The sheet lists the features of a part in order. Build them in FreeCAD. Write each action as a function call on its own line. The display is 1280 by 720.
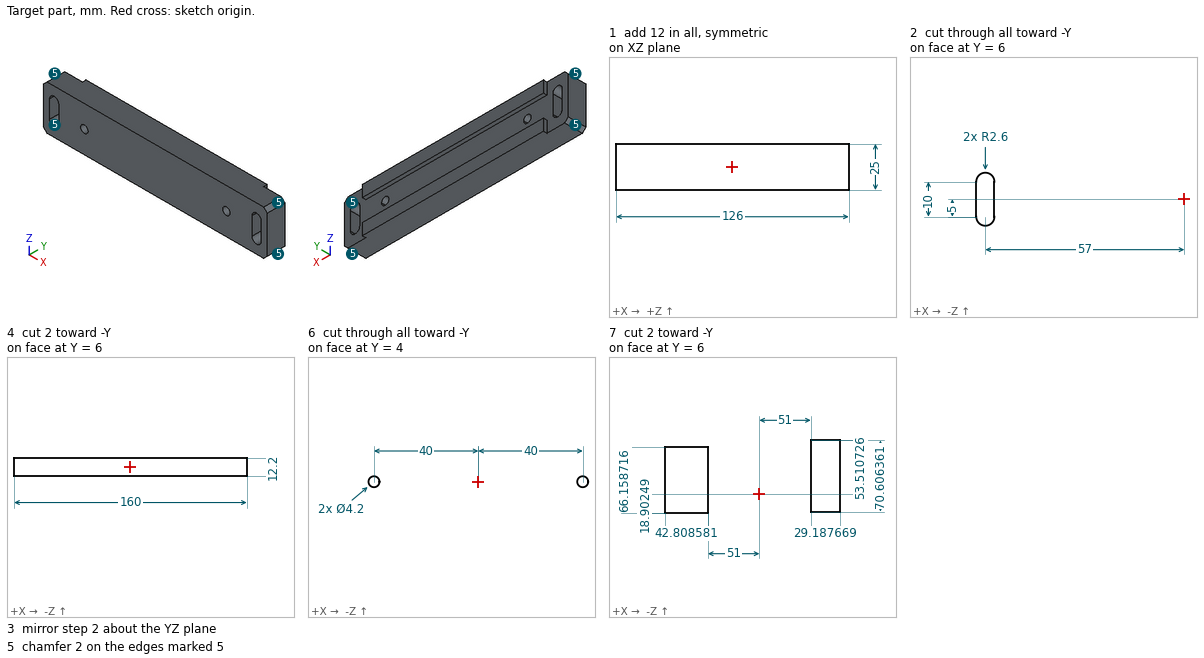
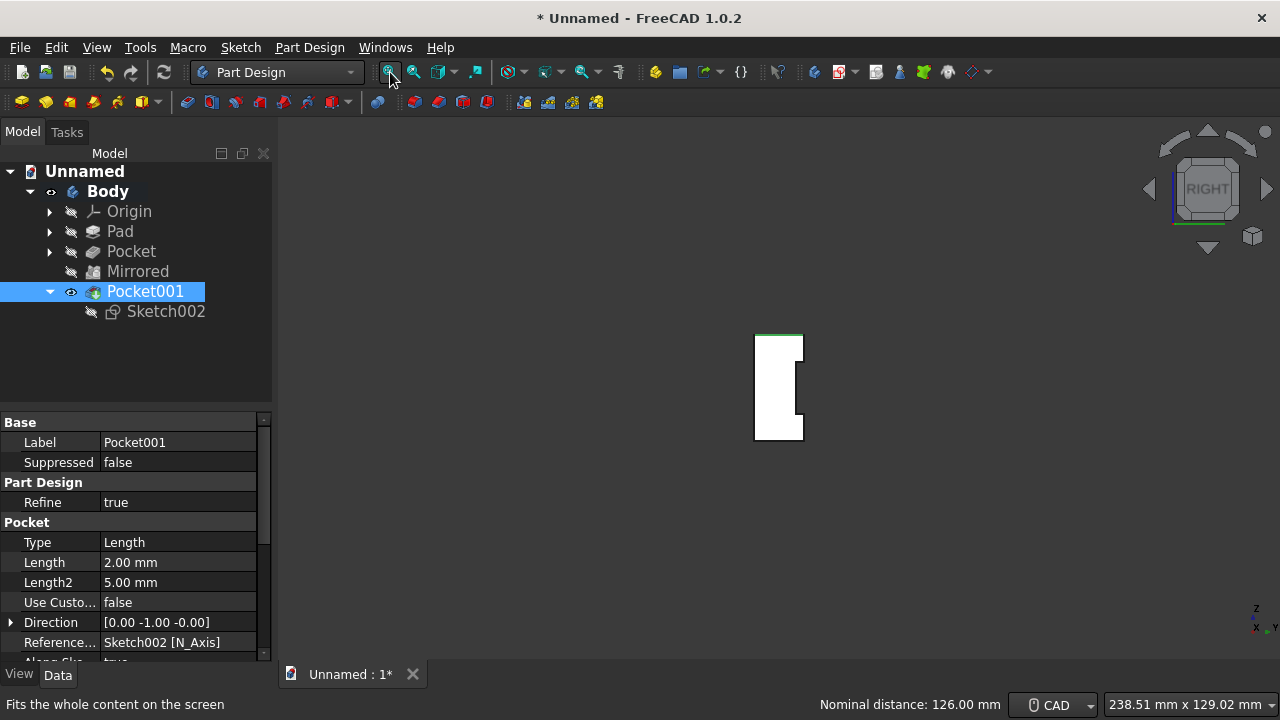
click(779, 440, ctrl)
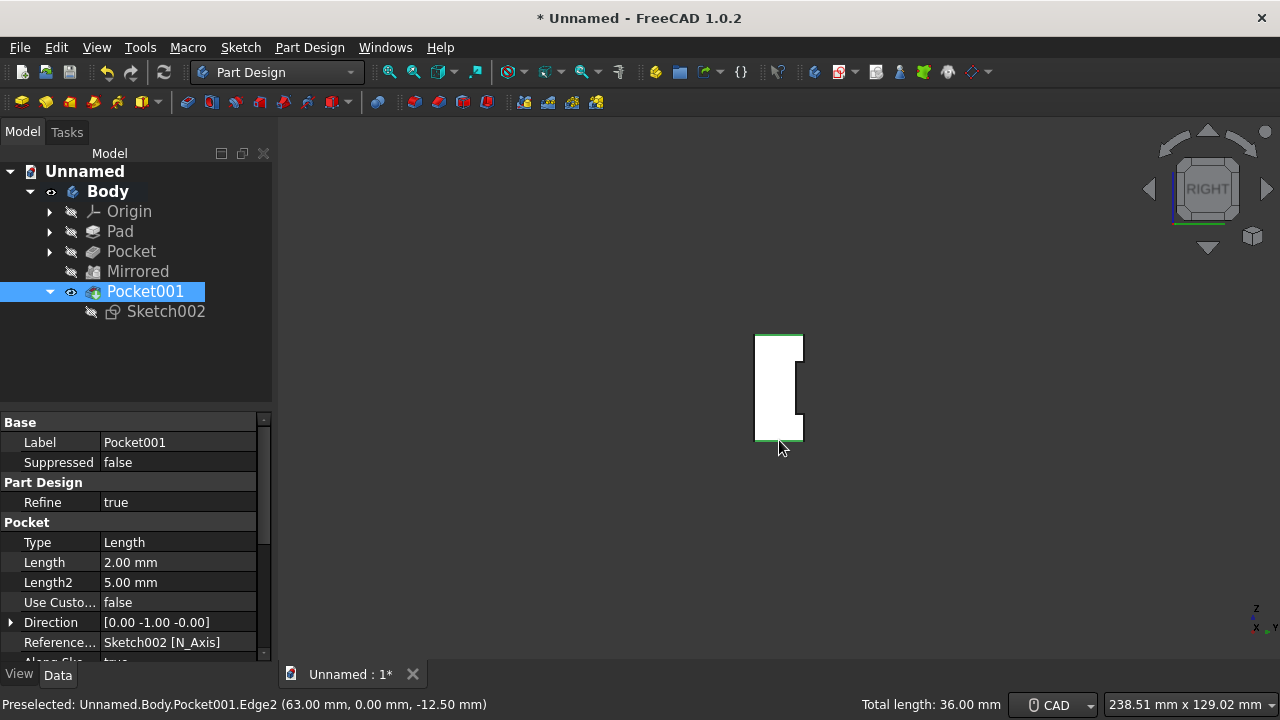
key(5)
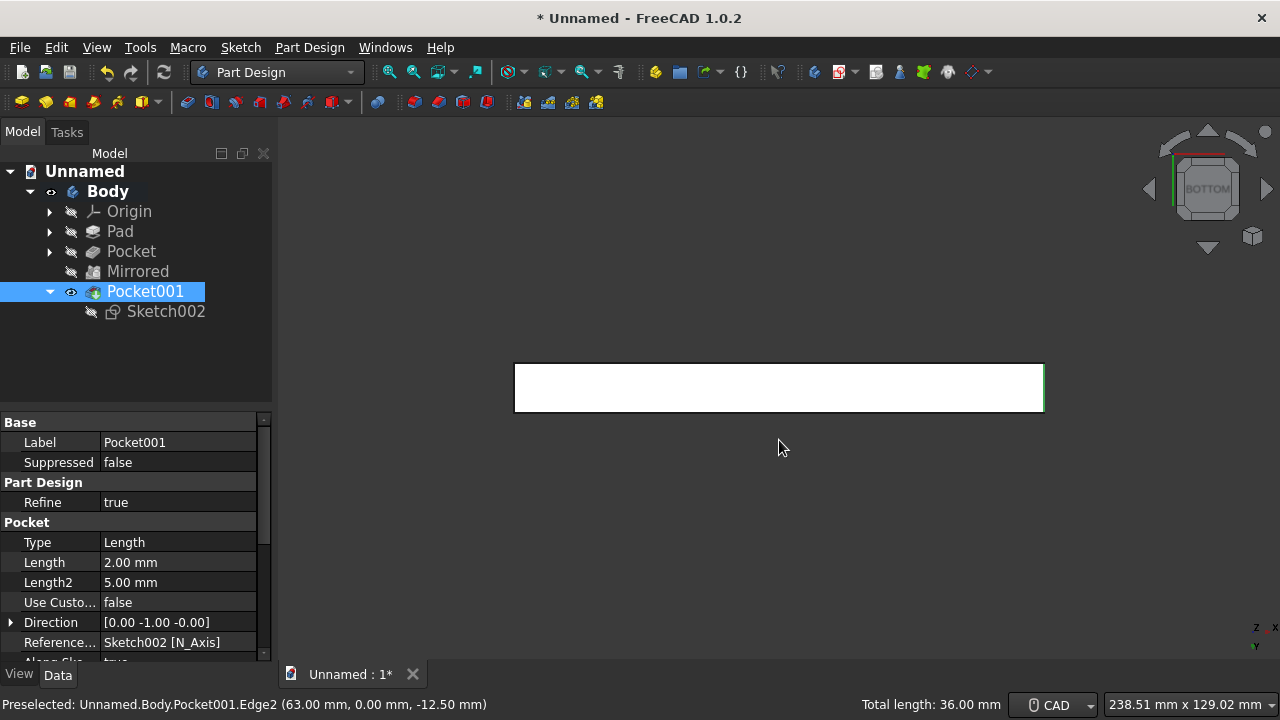
click(514, 387, ctrl)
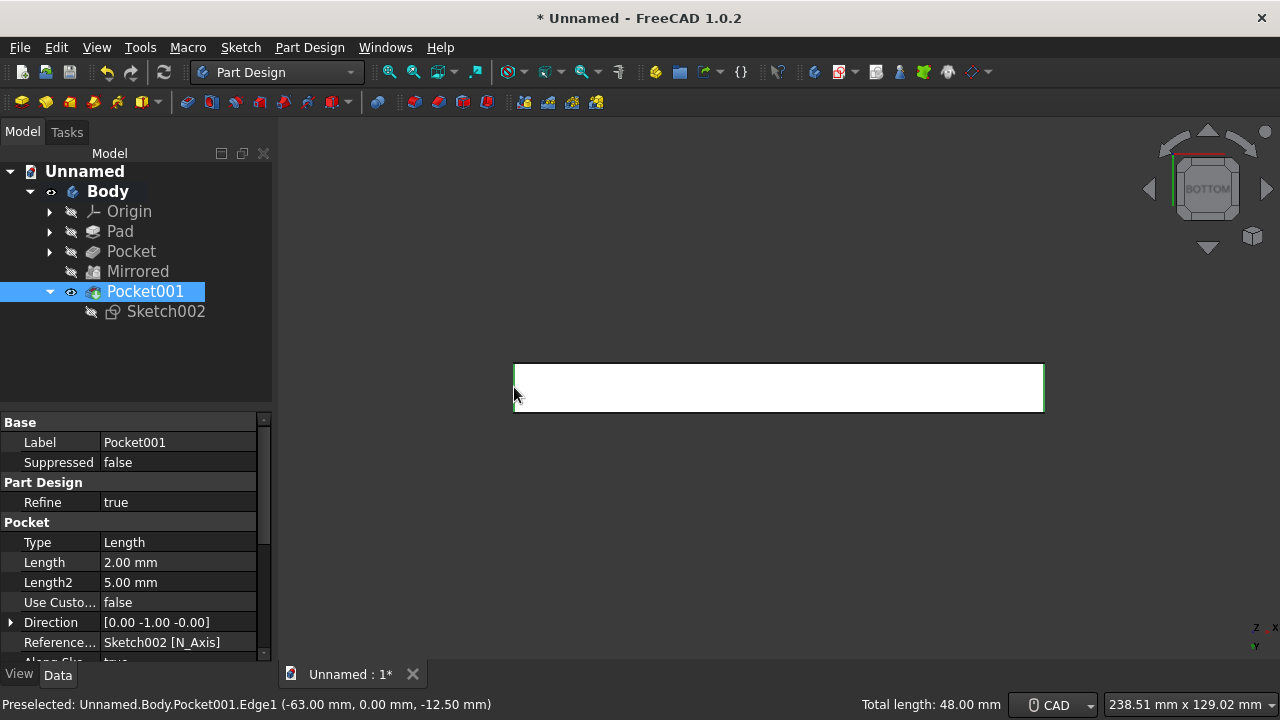
click(440, 102)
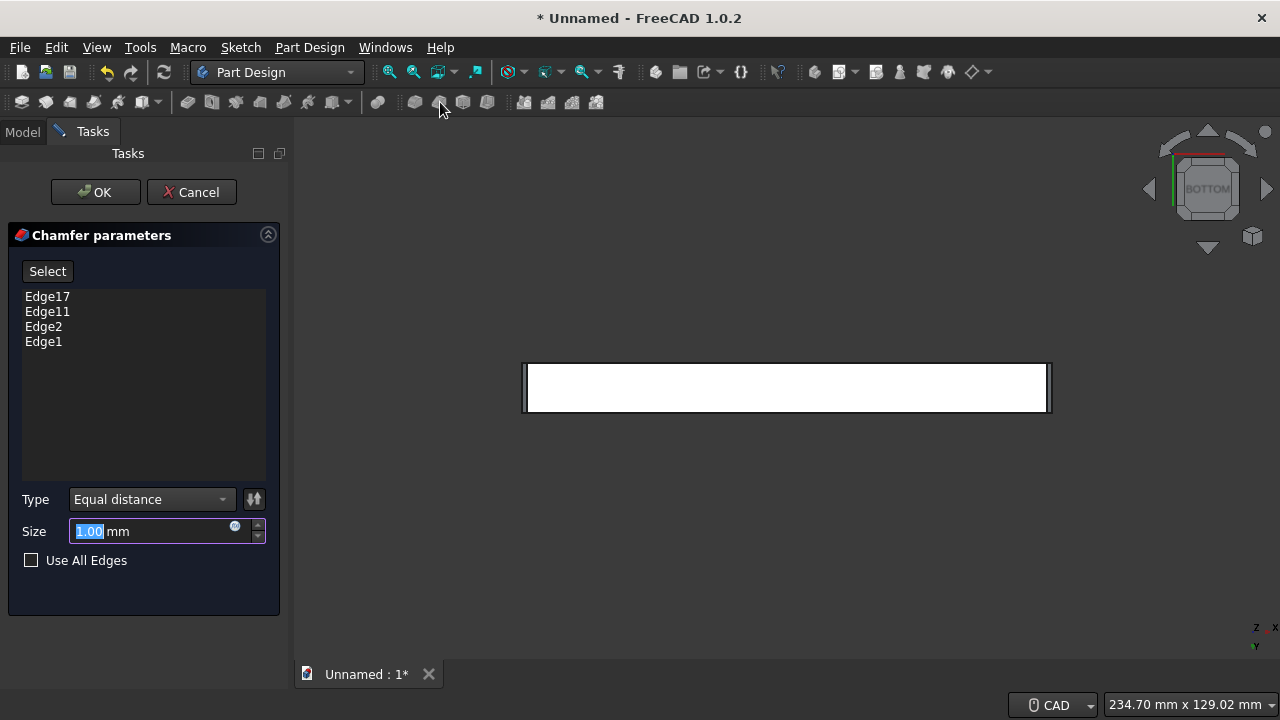
text(2)
key(Tab)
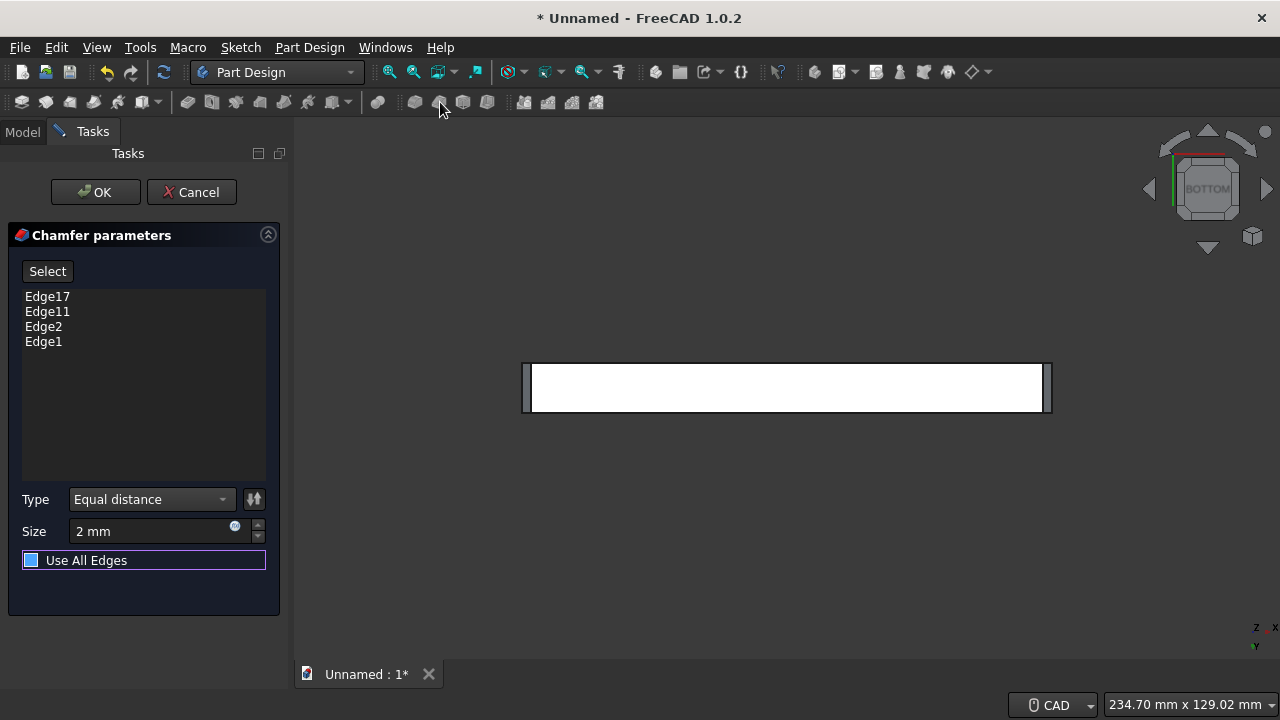
click(96, 192)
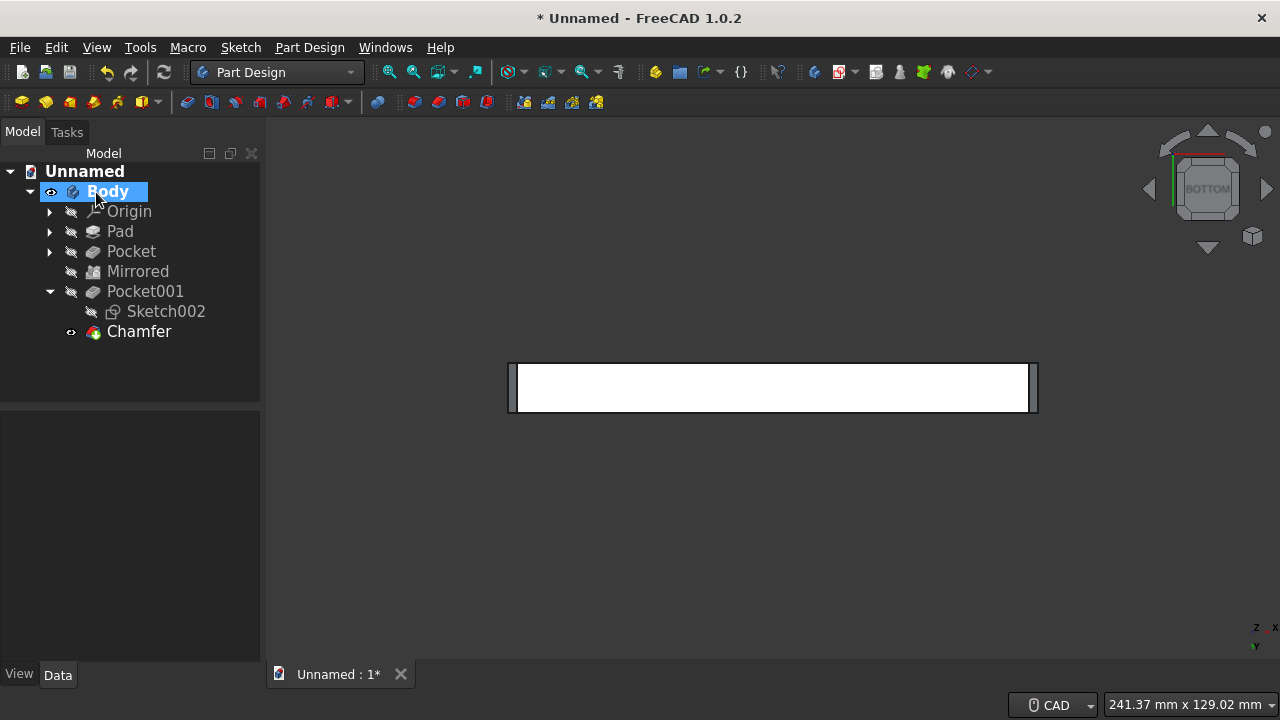
key(4)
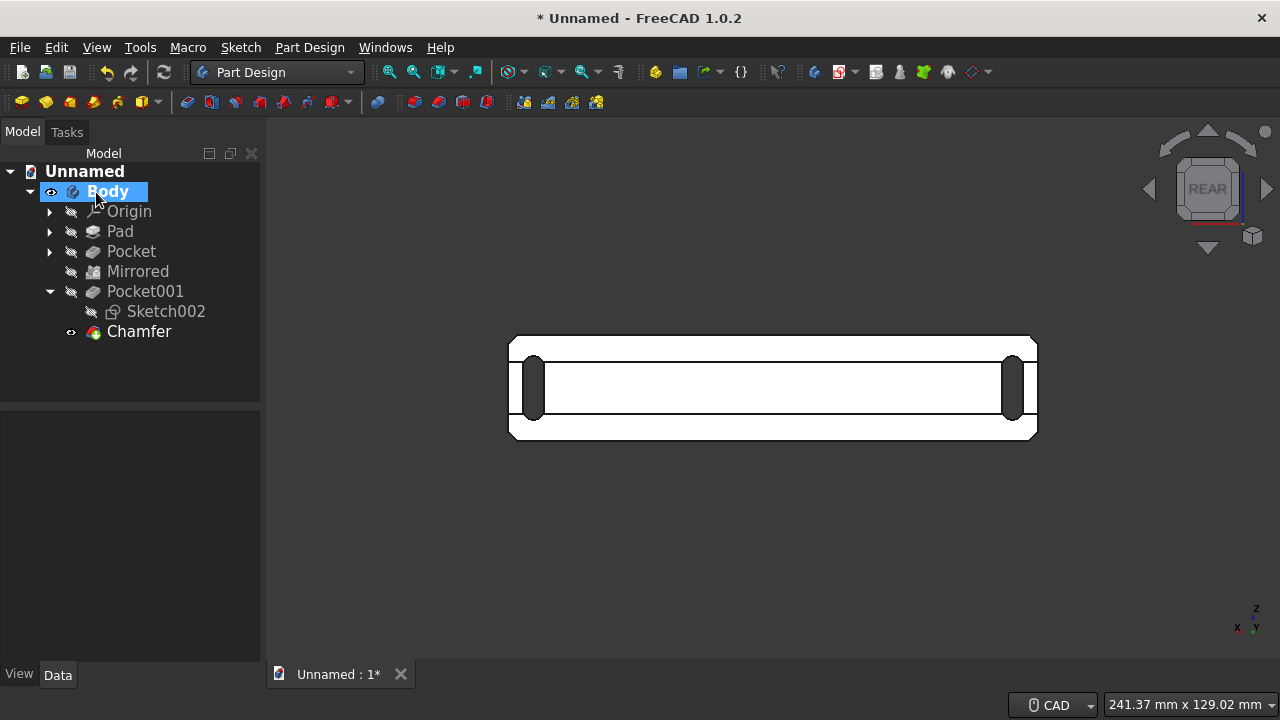
click(576, 387)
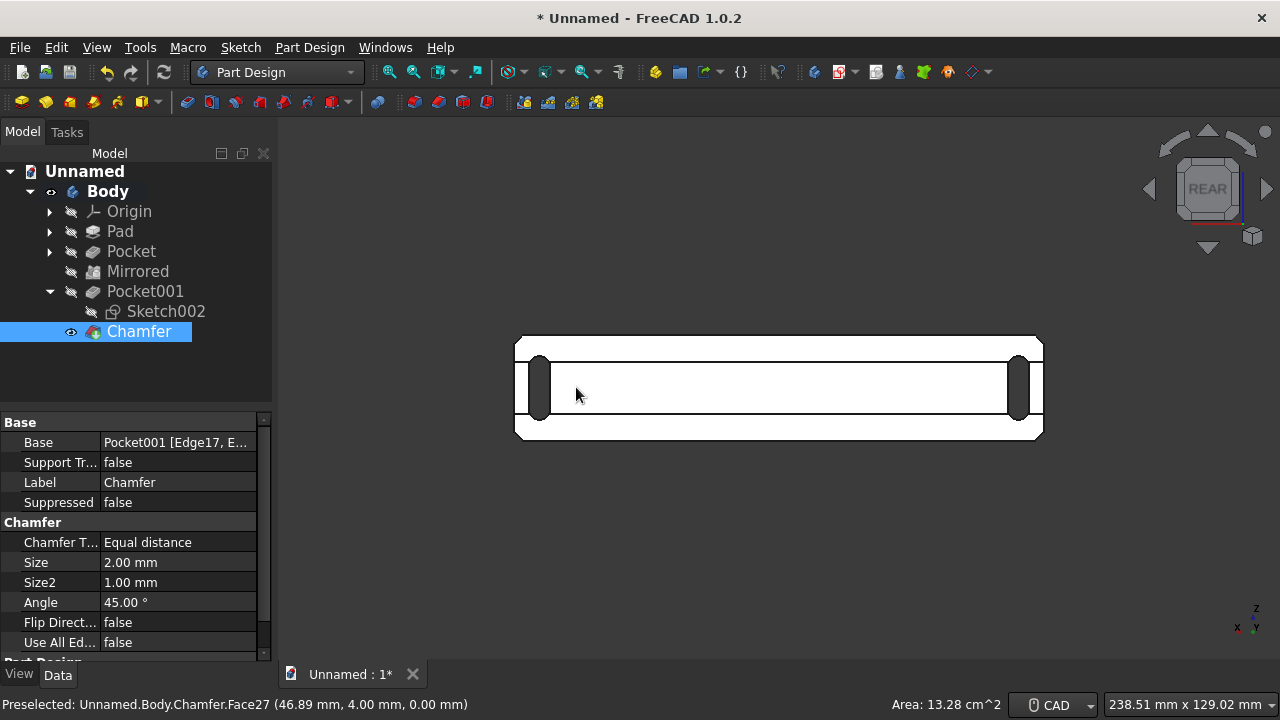
click(840, 72)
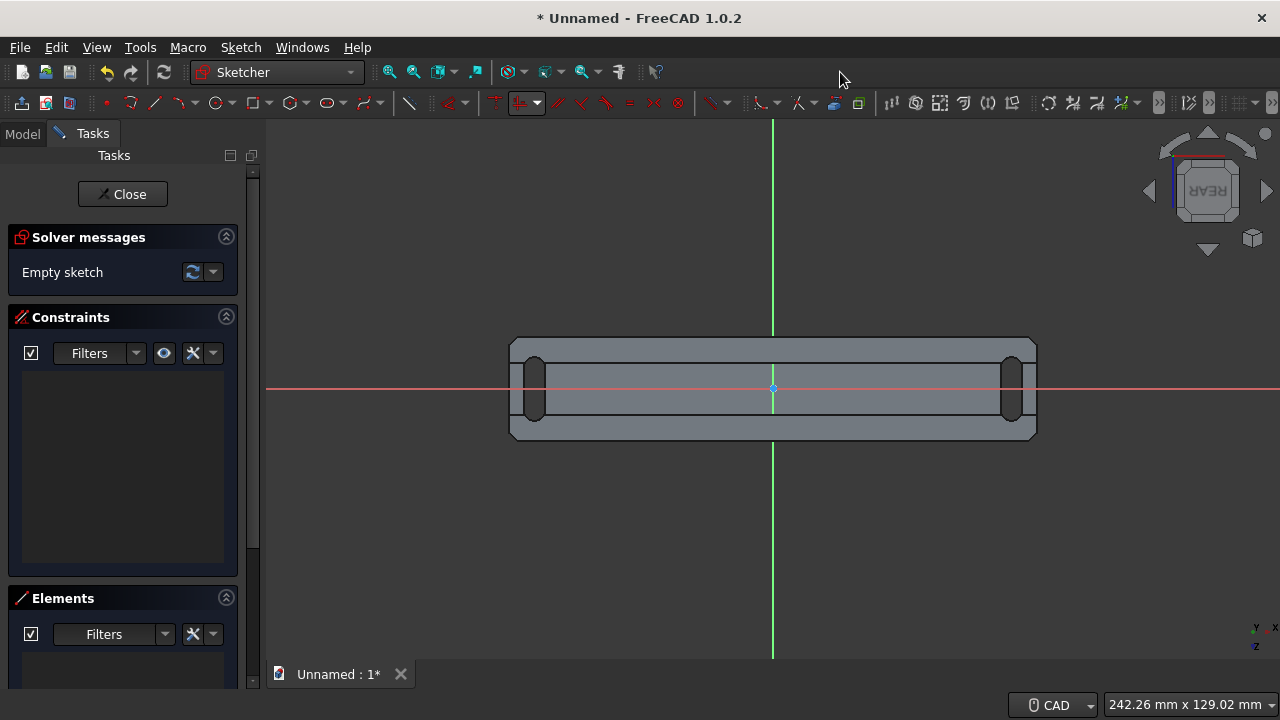
scroll(912, 389, up, 2)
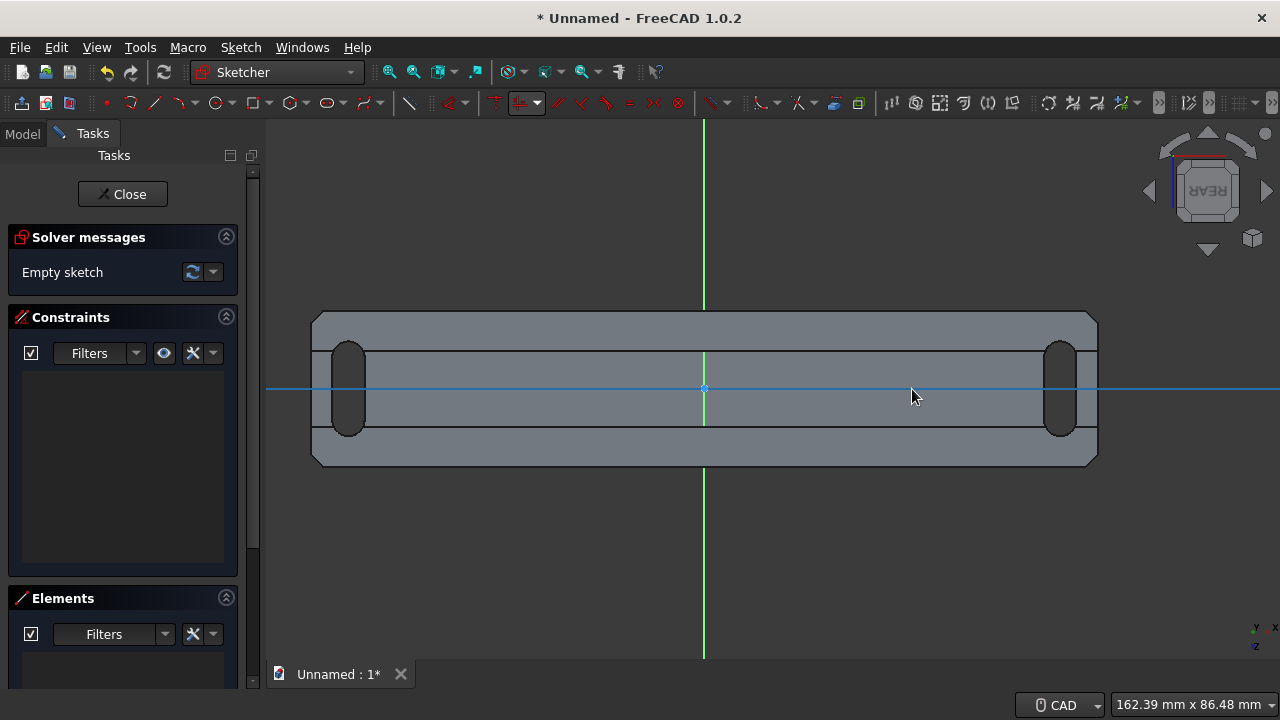
click(216, 104)